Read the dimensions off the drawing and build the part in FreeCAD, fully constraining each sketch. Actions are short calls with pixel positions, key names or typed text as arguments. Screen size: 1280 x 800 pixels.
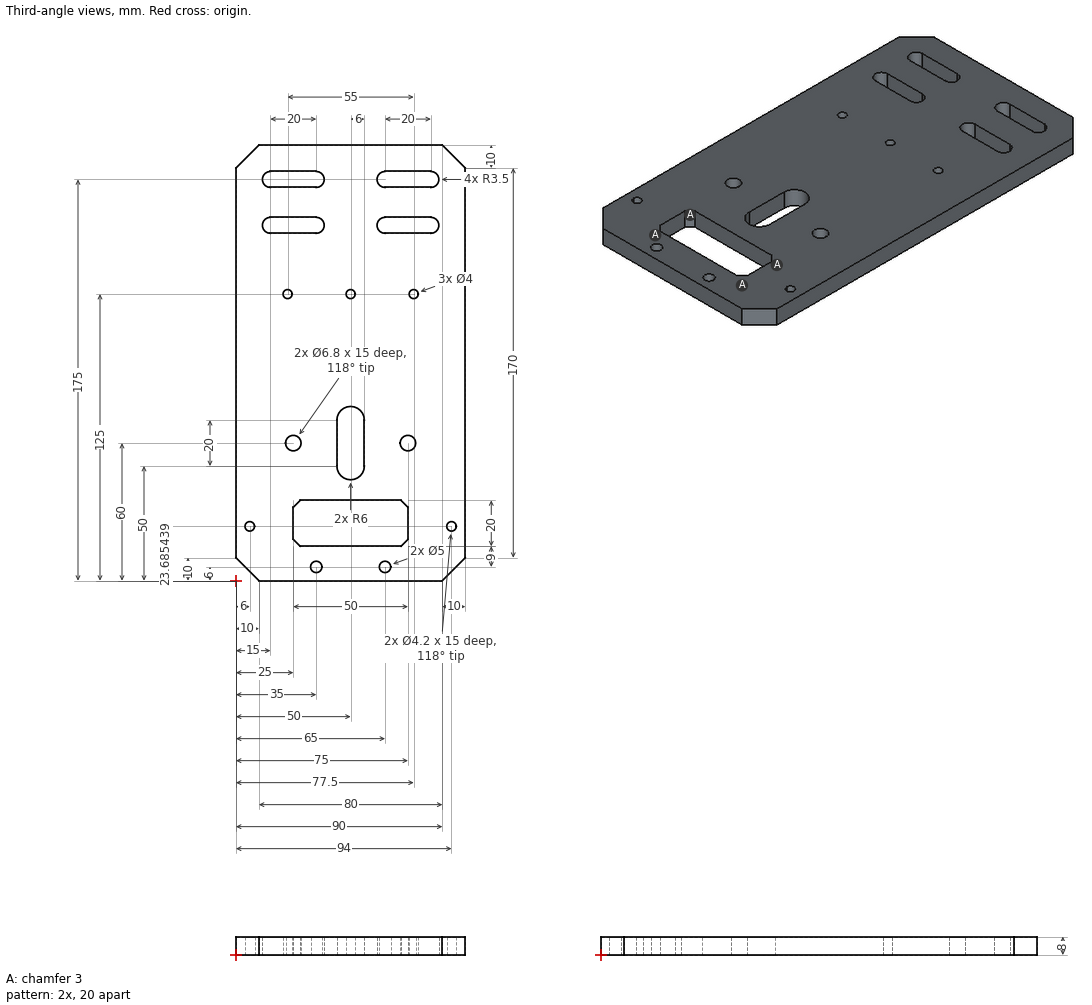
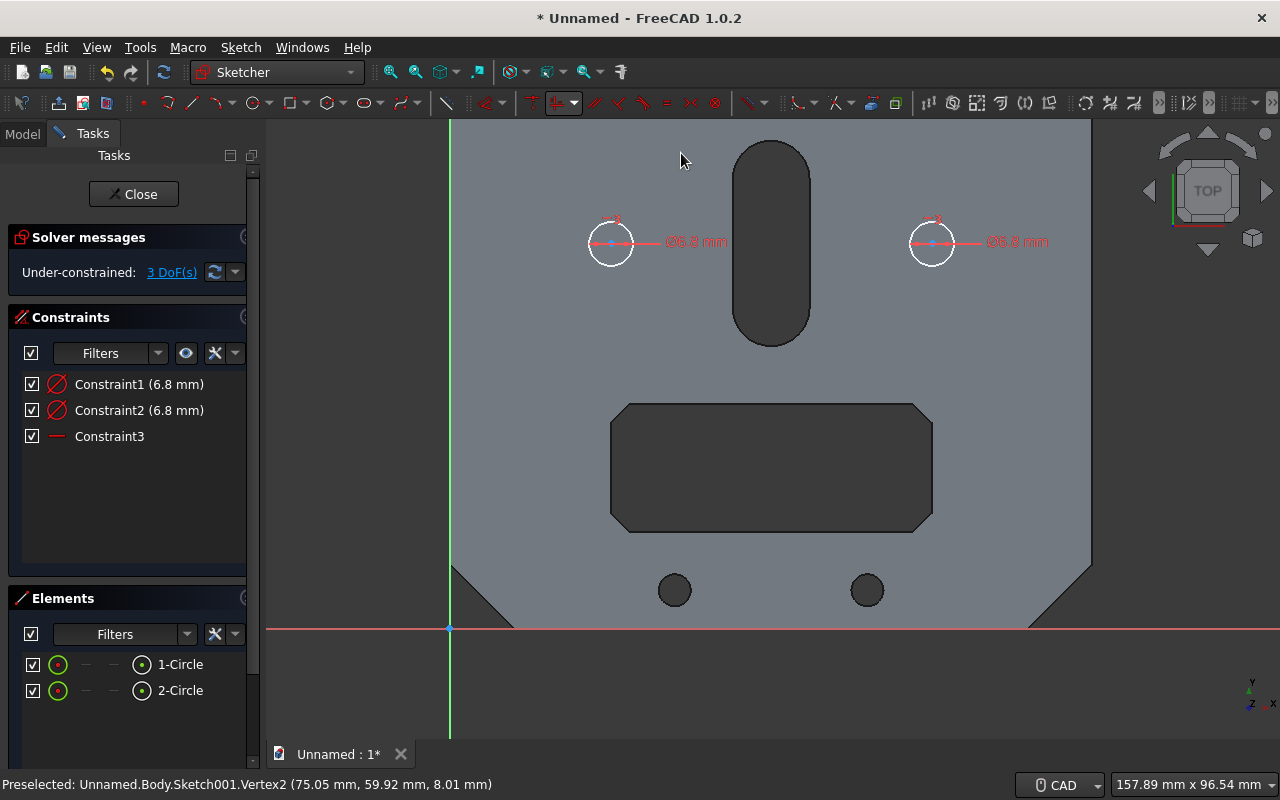
click(486, 104)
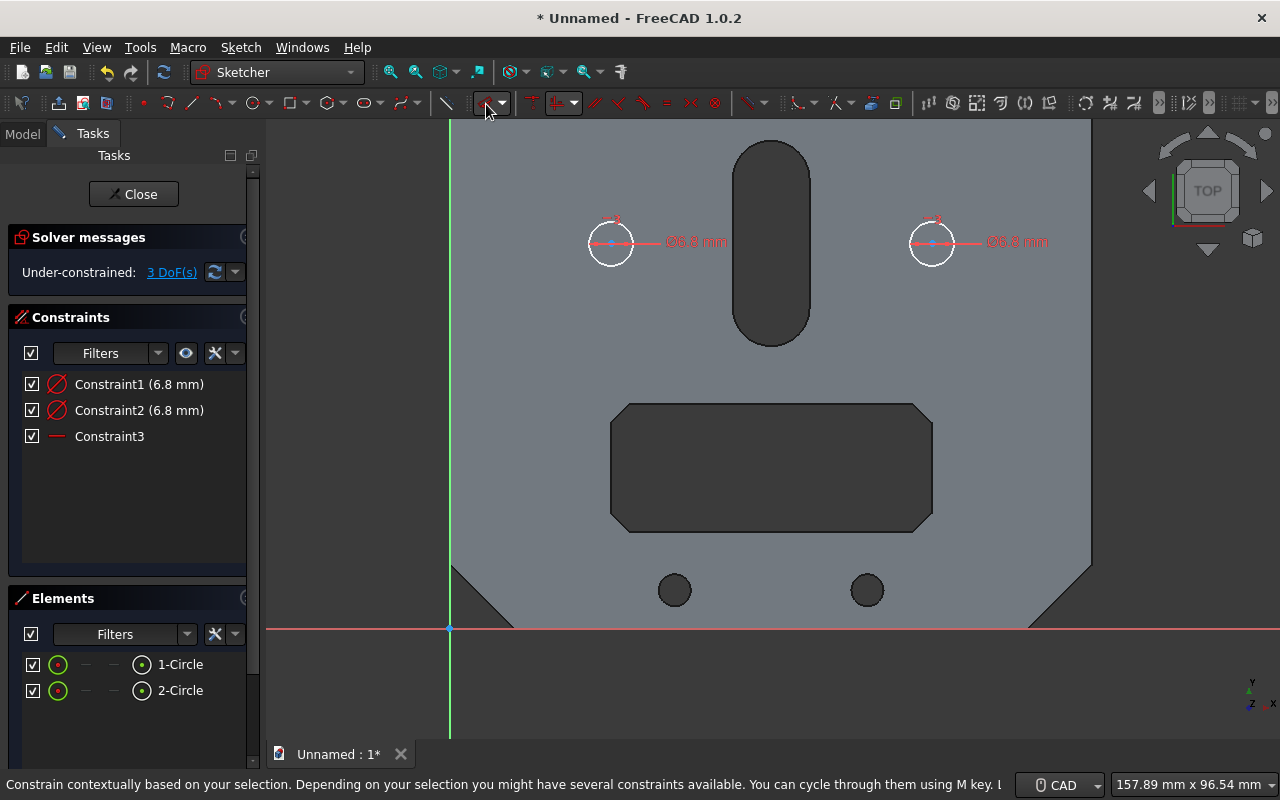
click(611, 244)
click(530, 663)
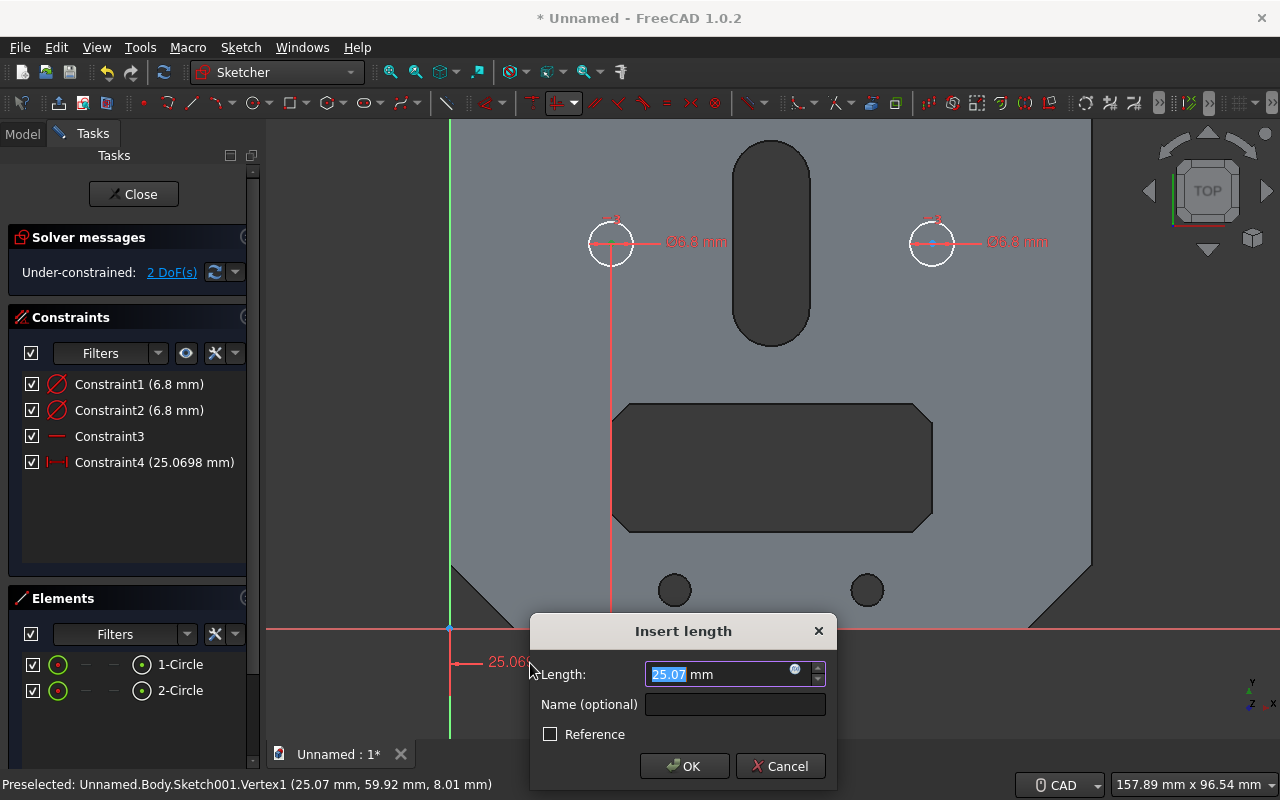
text(25)
key(Return)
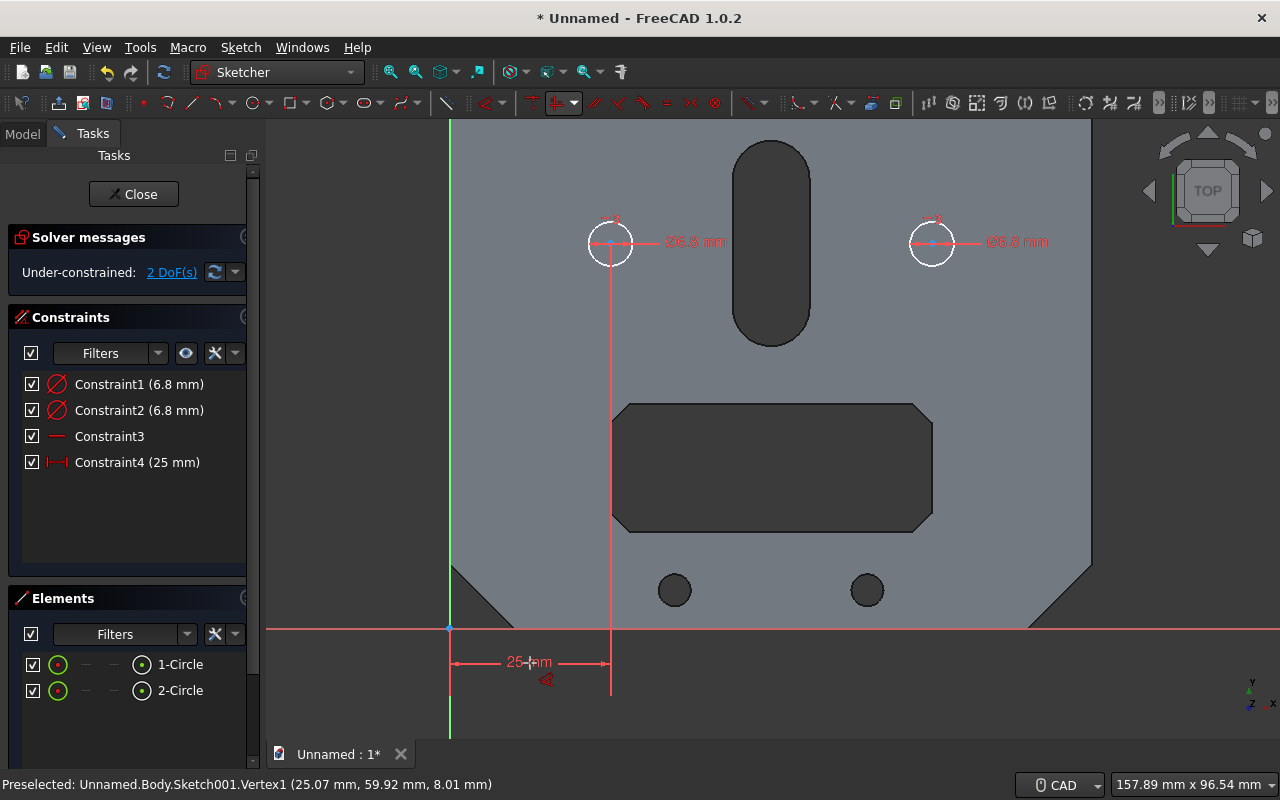
click(611, 244)
click(416, 436)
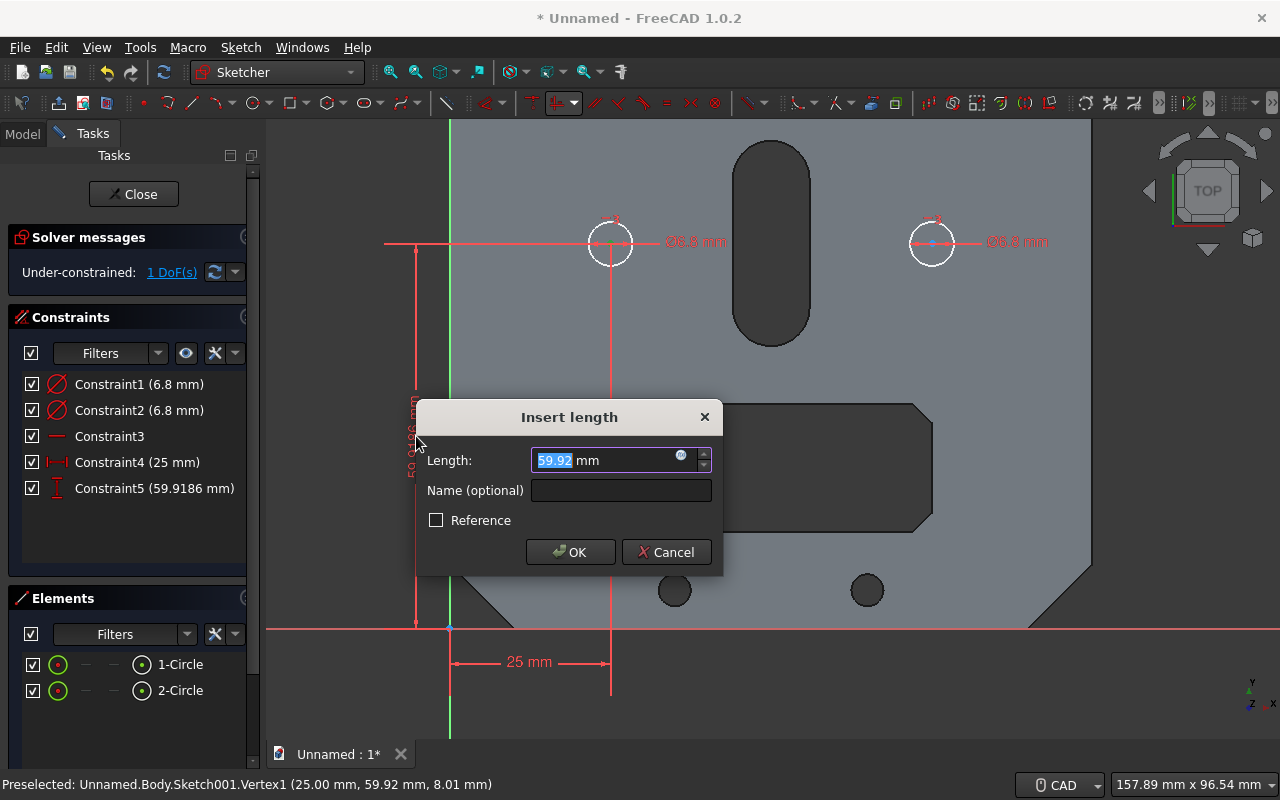
text(60)
key(Return)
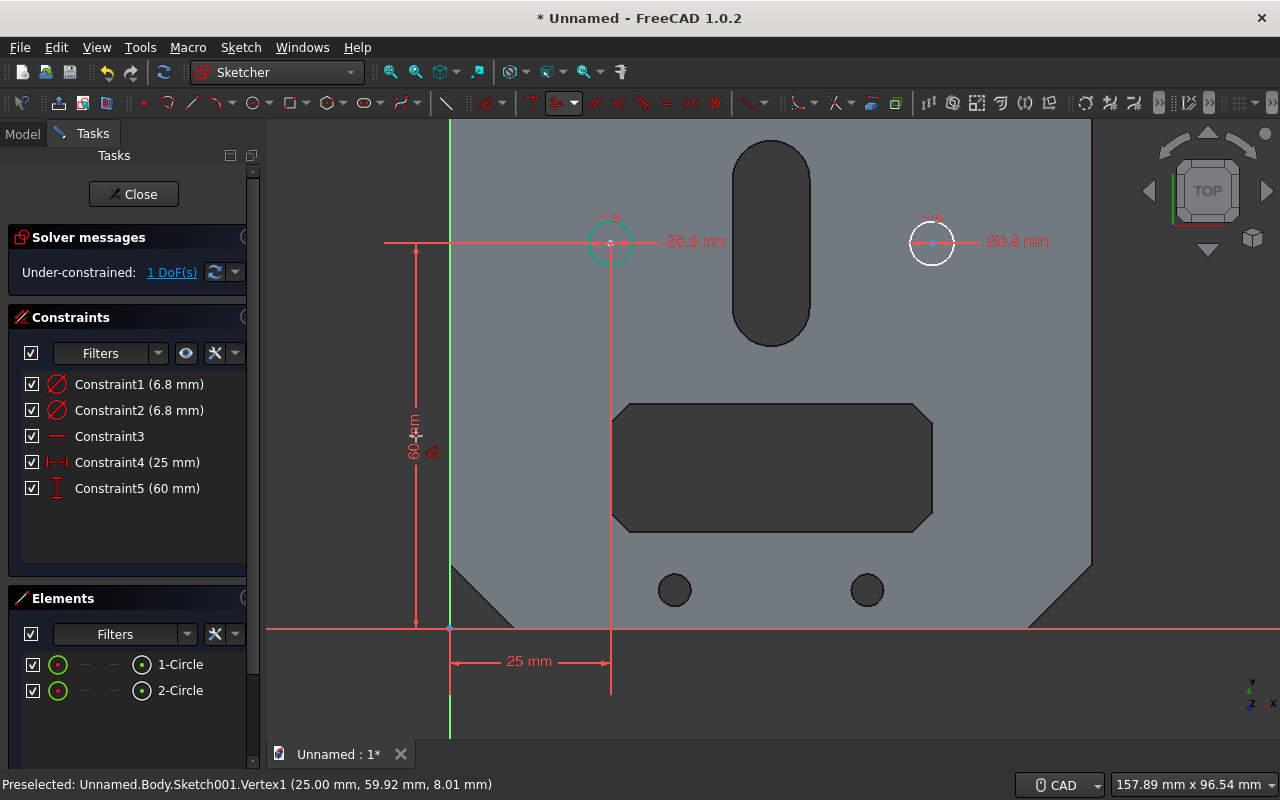
click(932, 243)
click(691, 663)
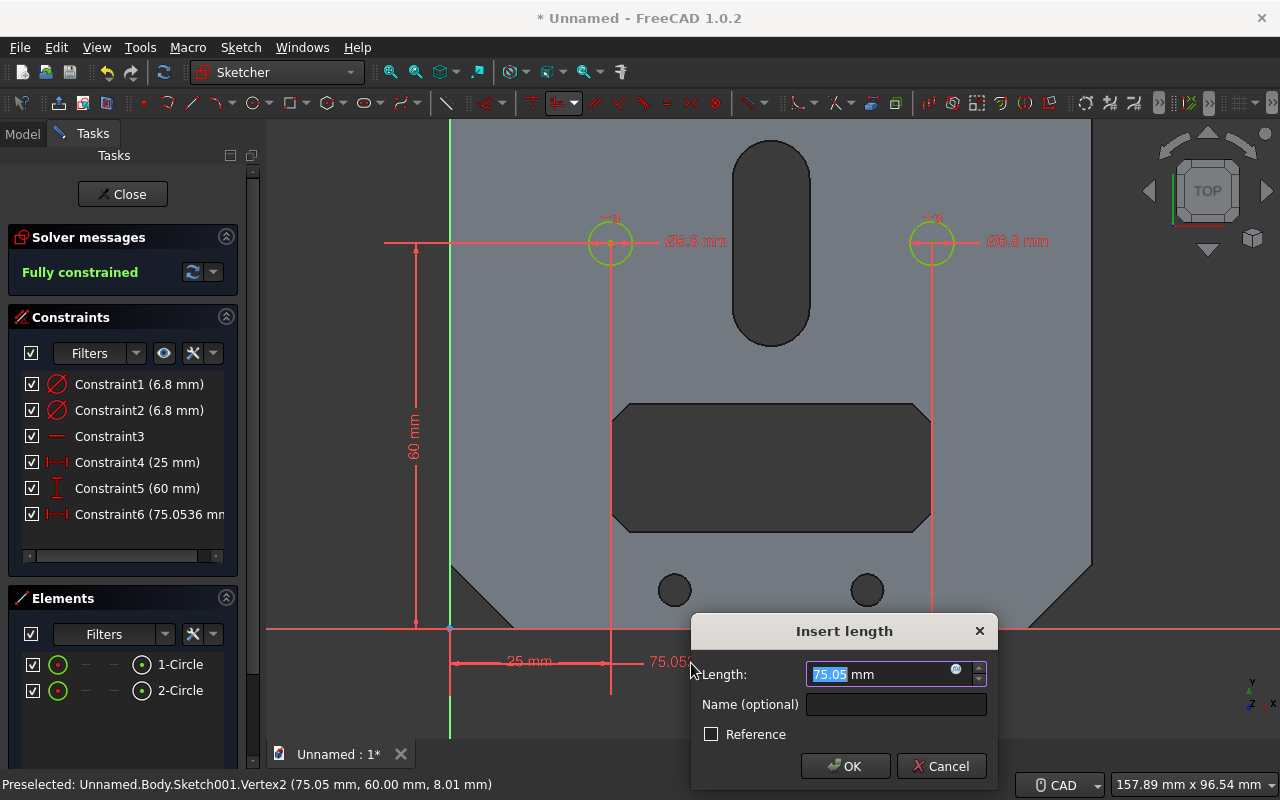
text(75)
key(Return)
key(Escape)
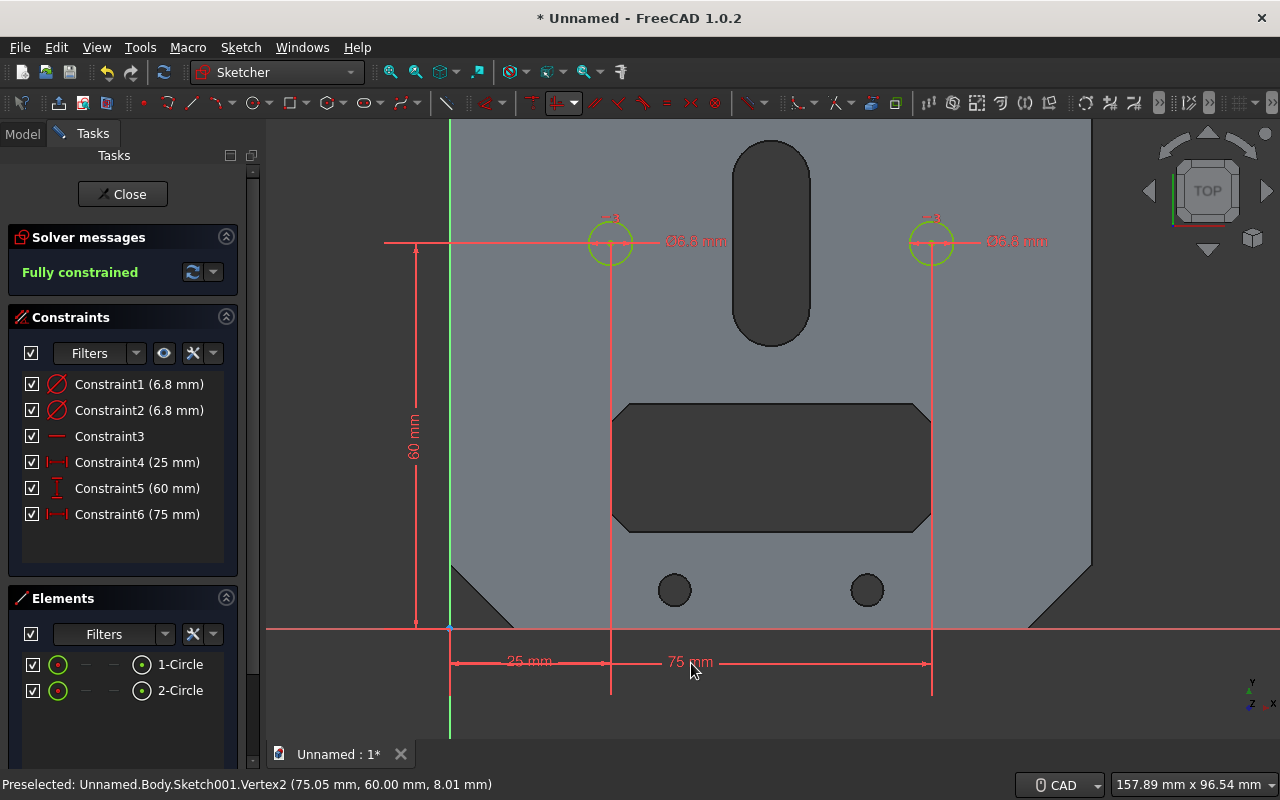
click(123, 194)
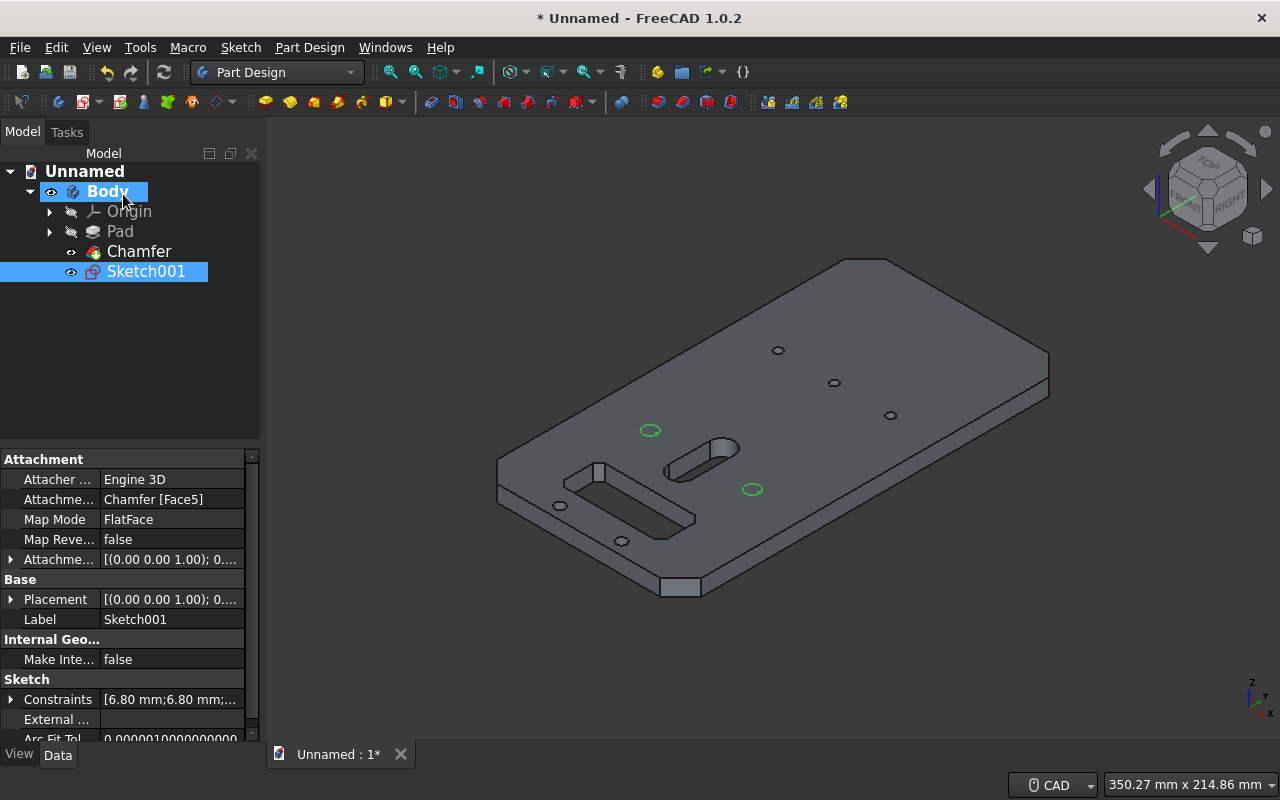
click(456, 102)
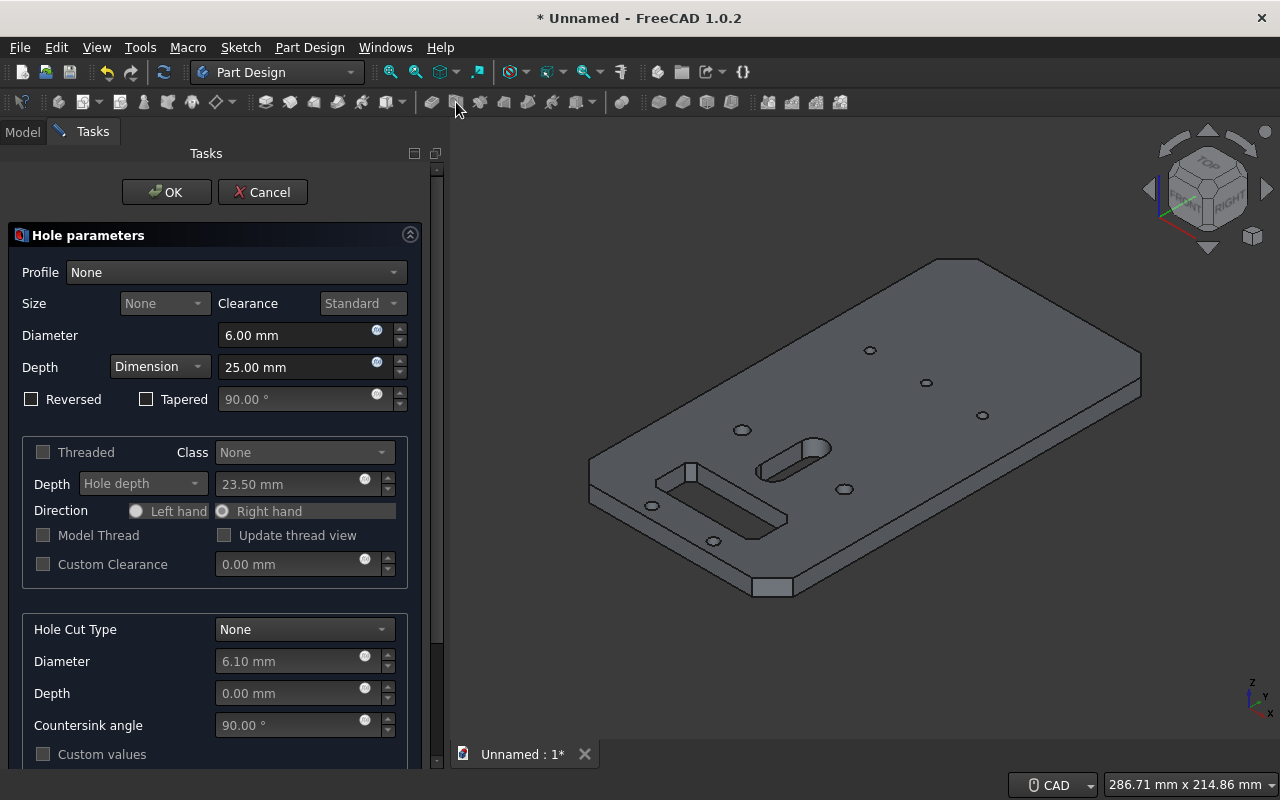
triple_click(305, 335)